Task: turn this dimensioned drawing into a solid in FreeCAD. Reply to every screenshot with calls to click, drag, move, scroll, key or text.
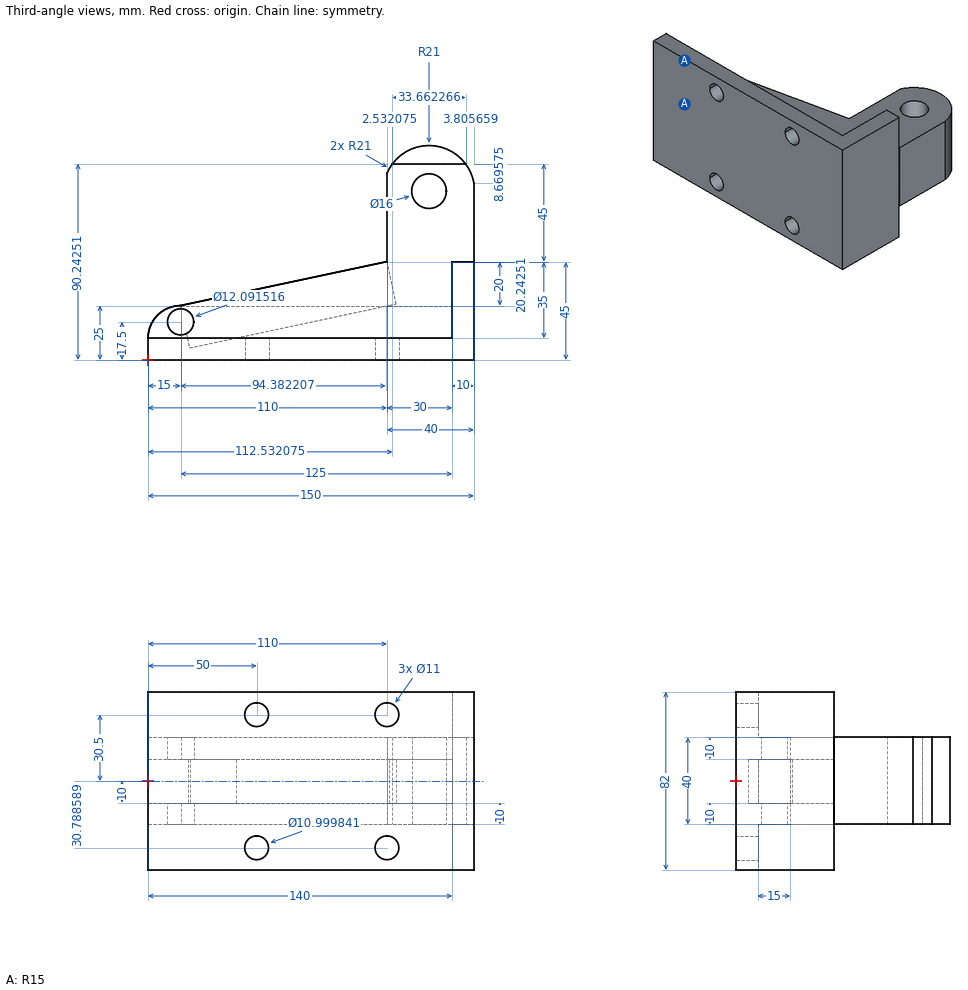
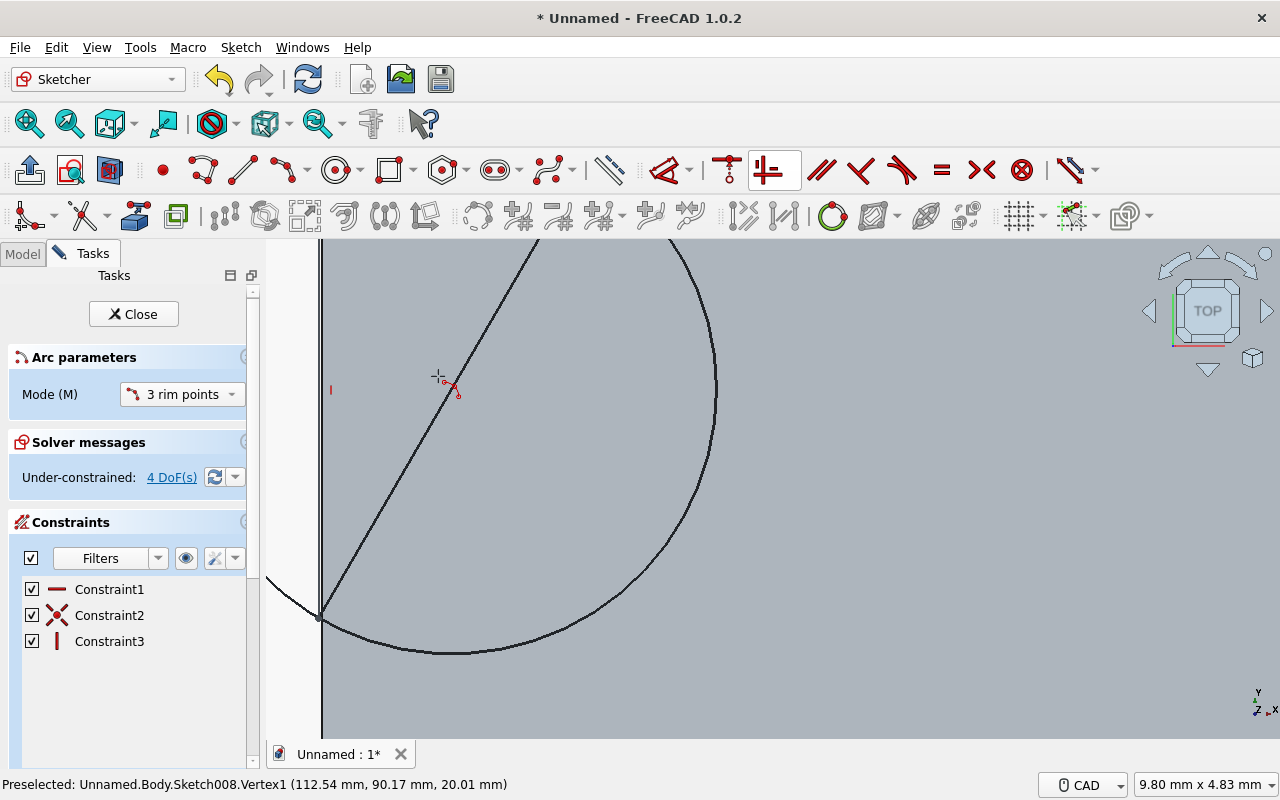
click(439, 374)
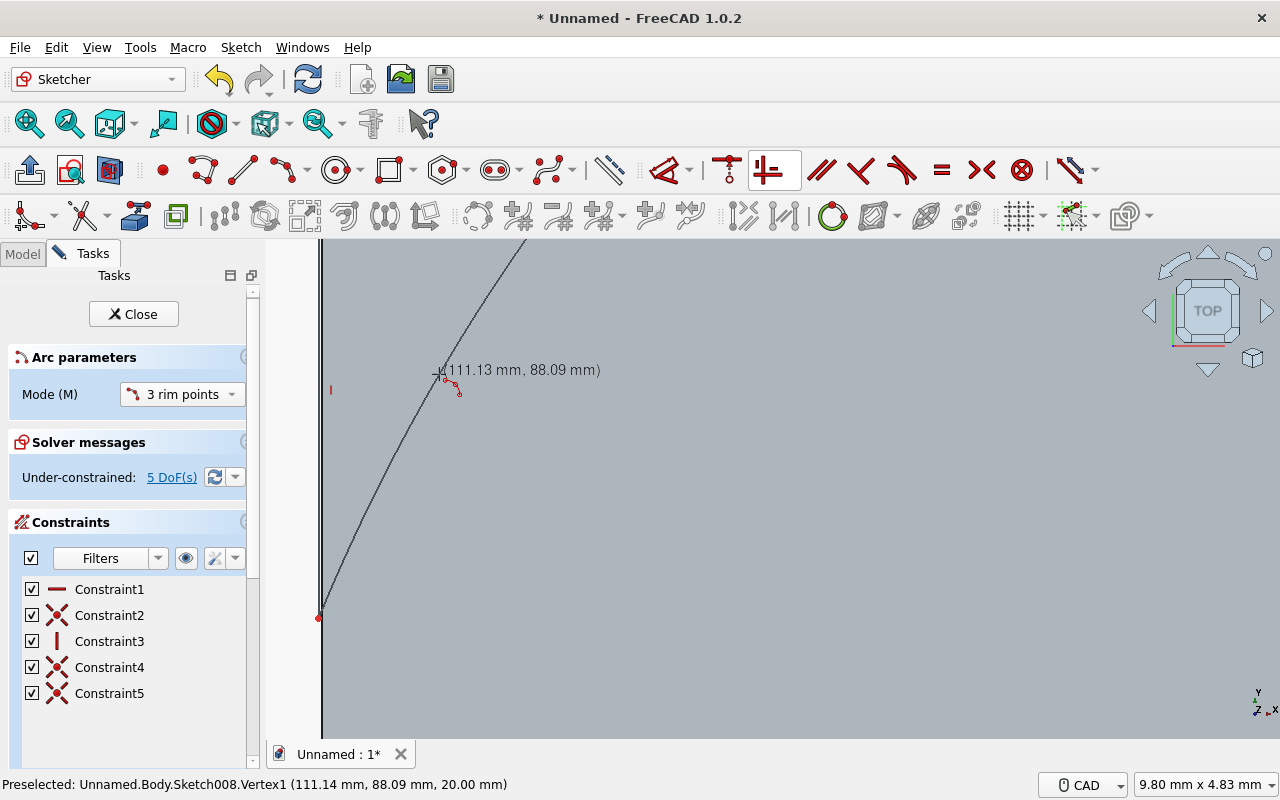
click(204, 170)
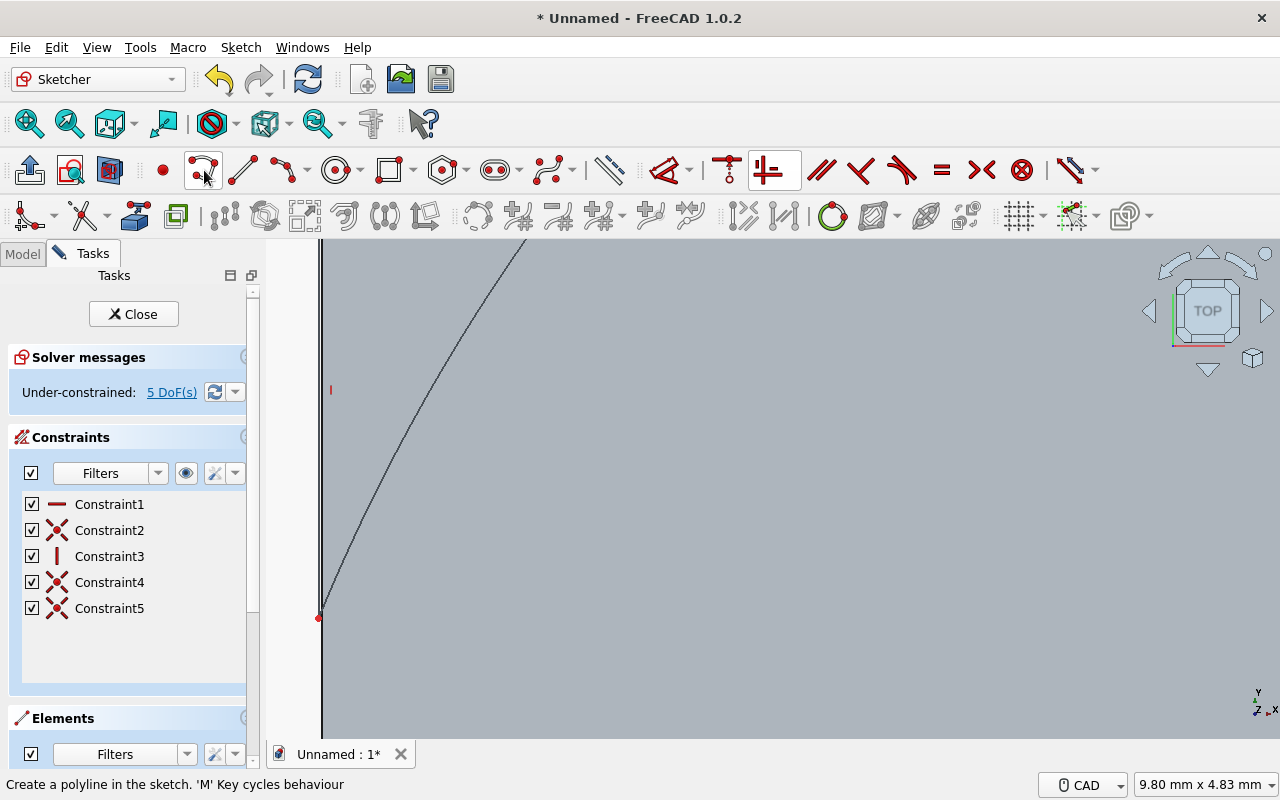
scroll(440, 375, down, 10)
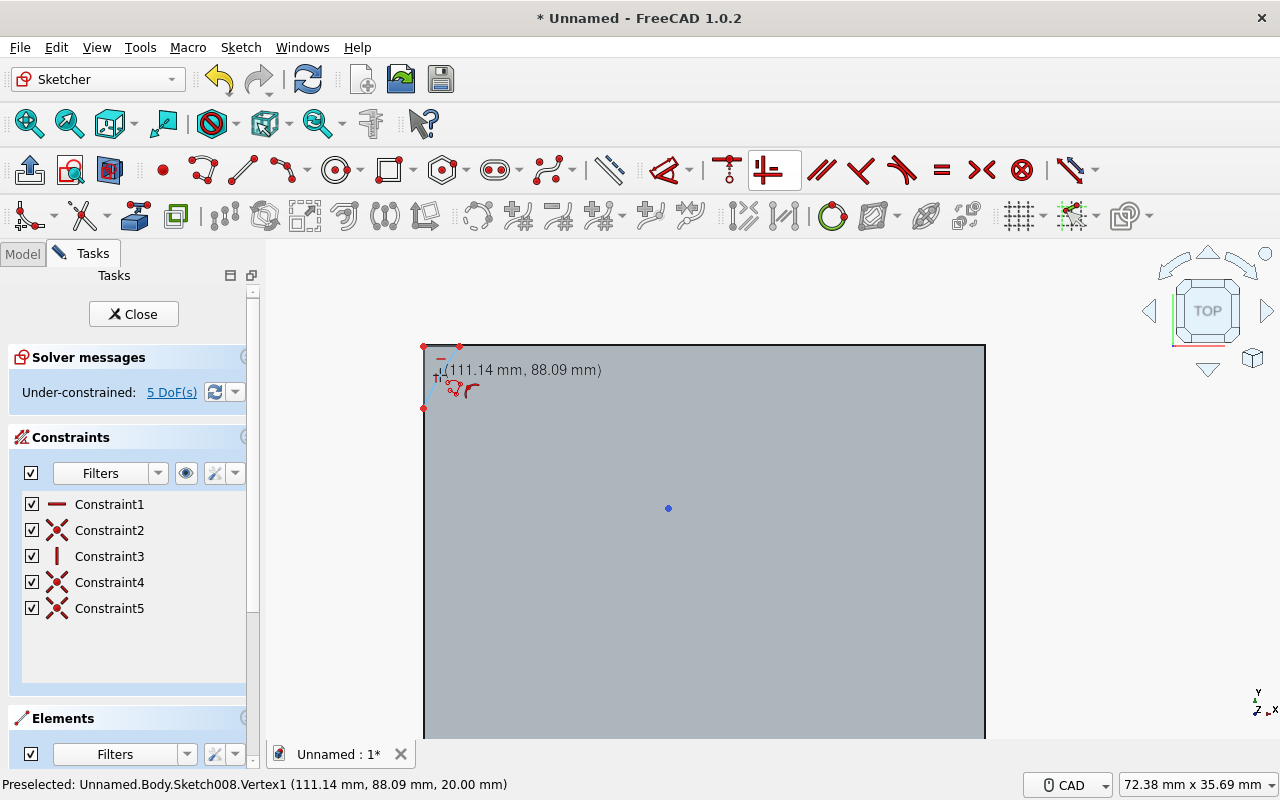
click(985, 467)
click(985, 345)
click(931, 345)
right_click(931, 345)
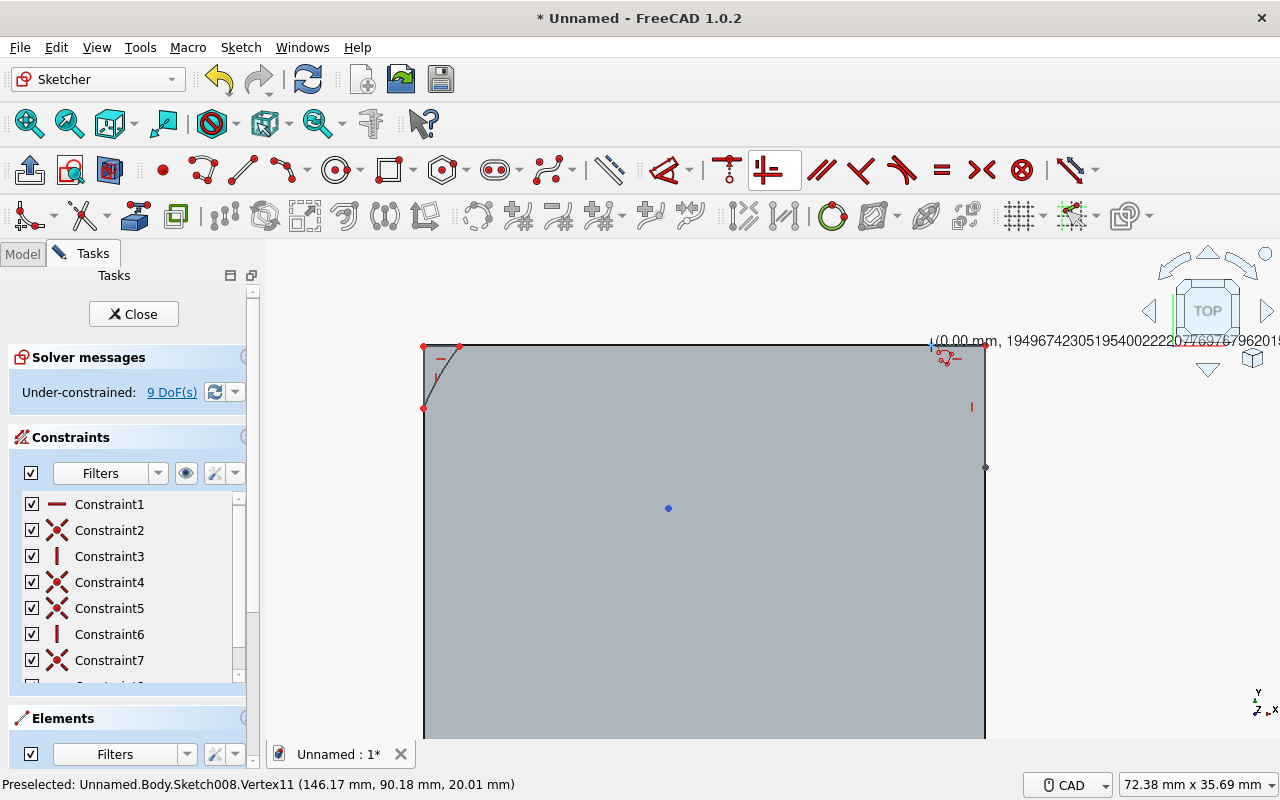
click(284, 170)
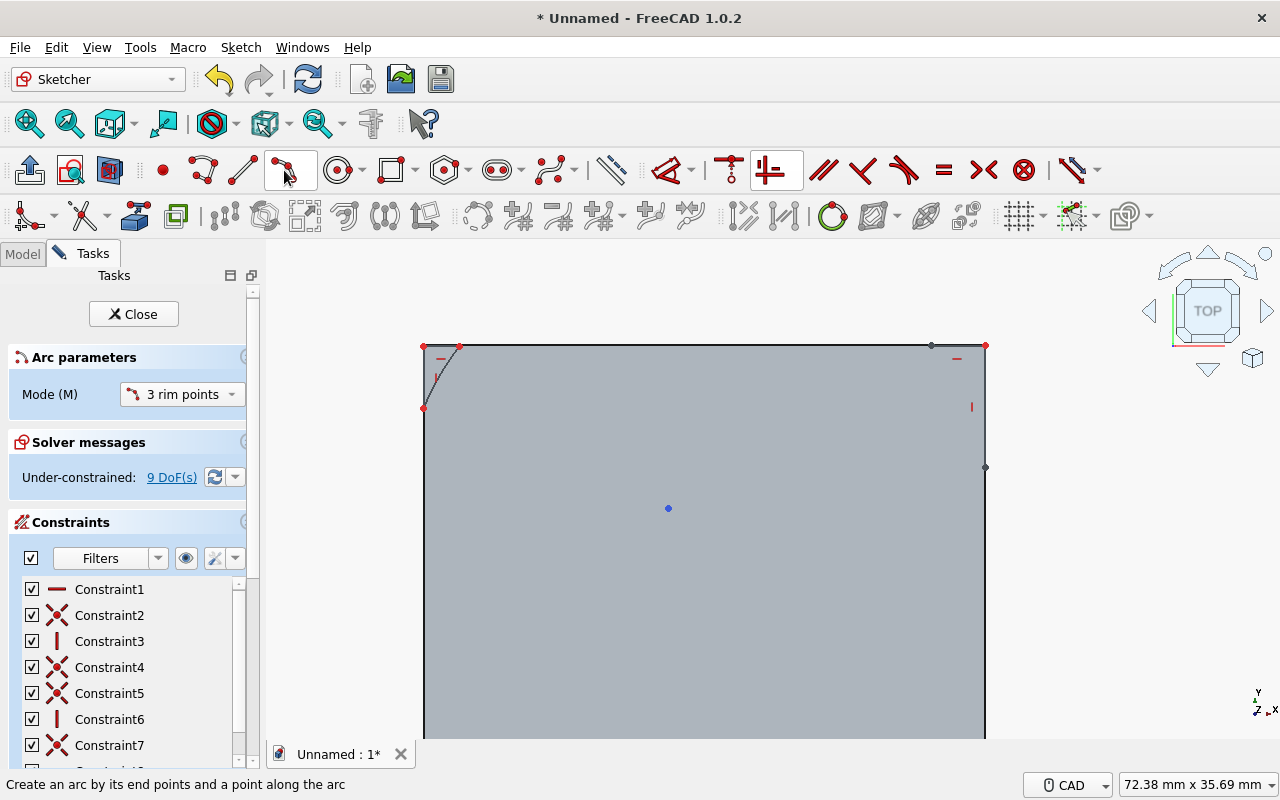
click(931, 346)
click(985, 468)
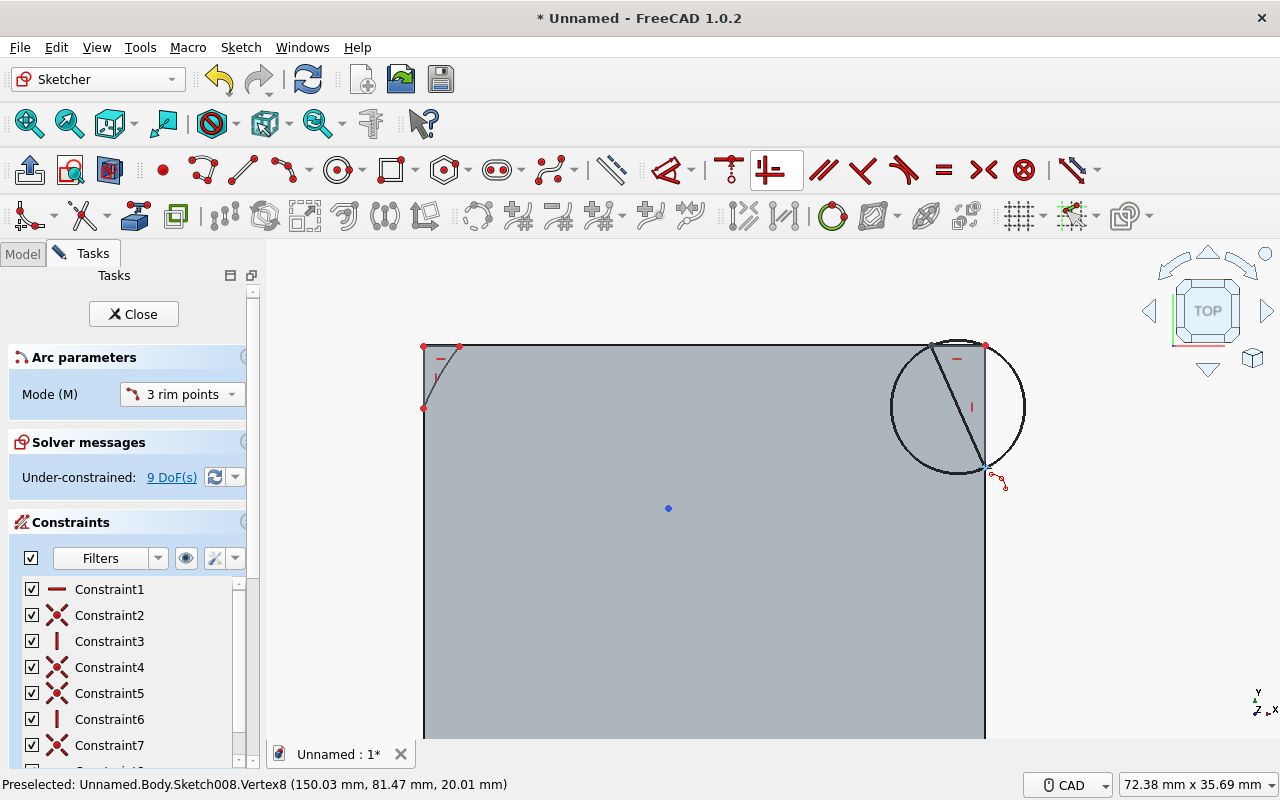
scroll(965, 403, up, 4)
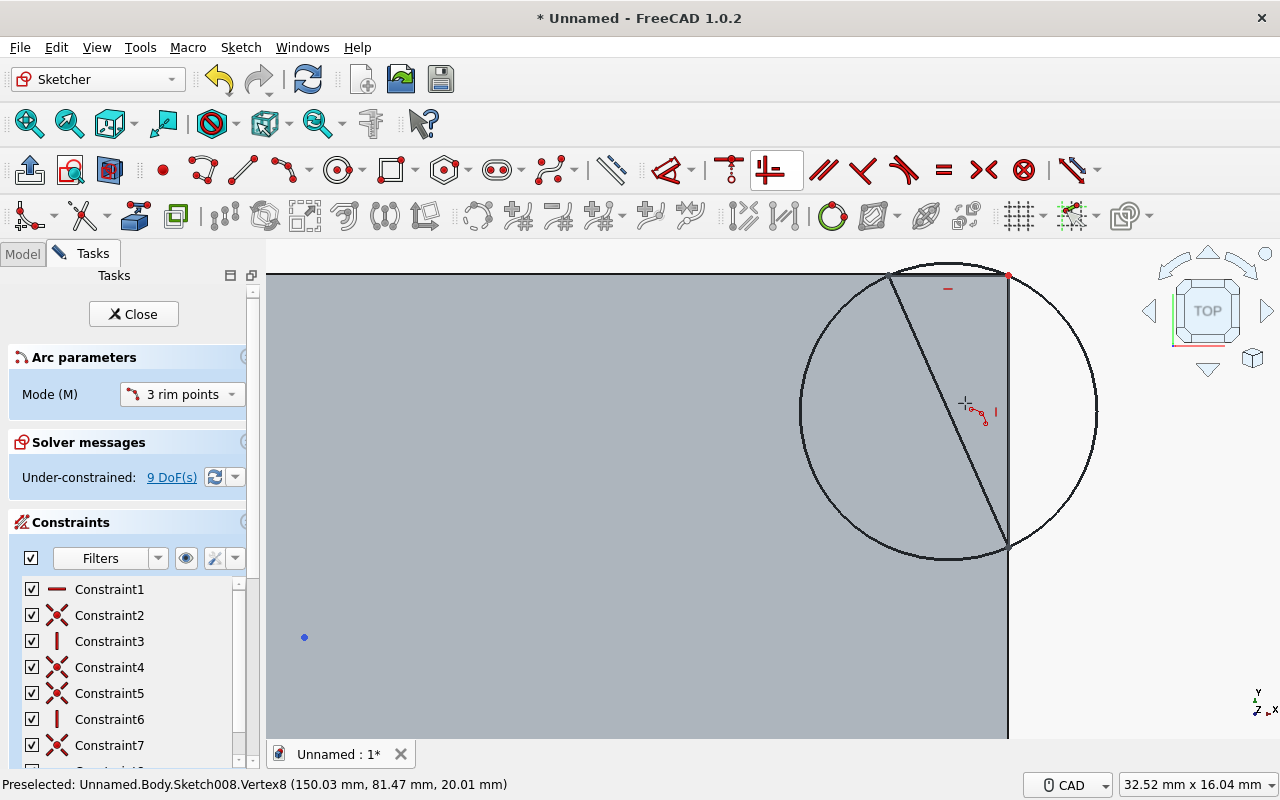
click(964, 402)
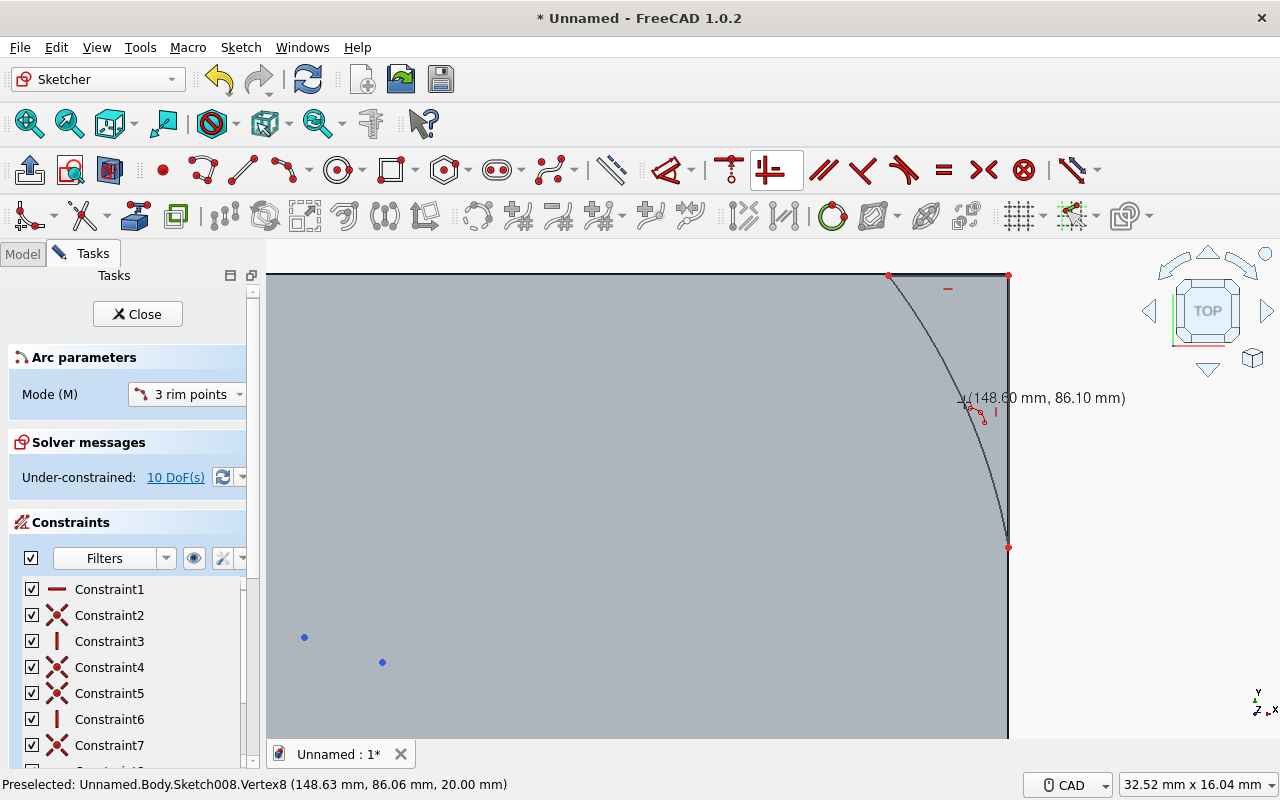
key(g)
key(c)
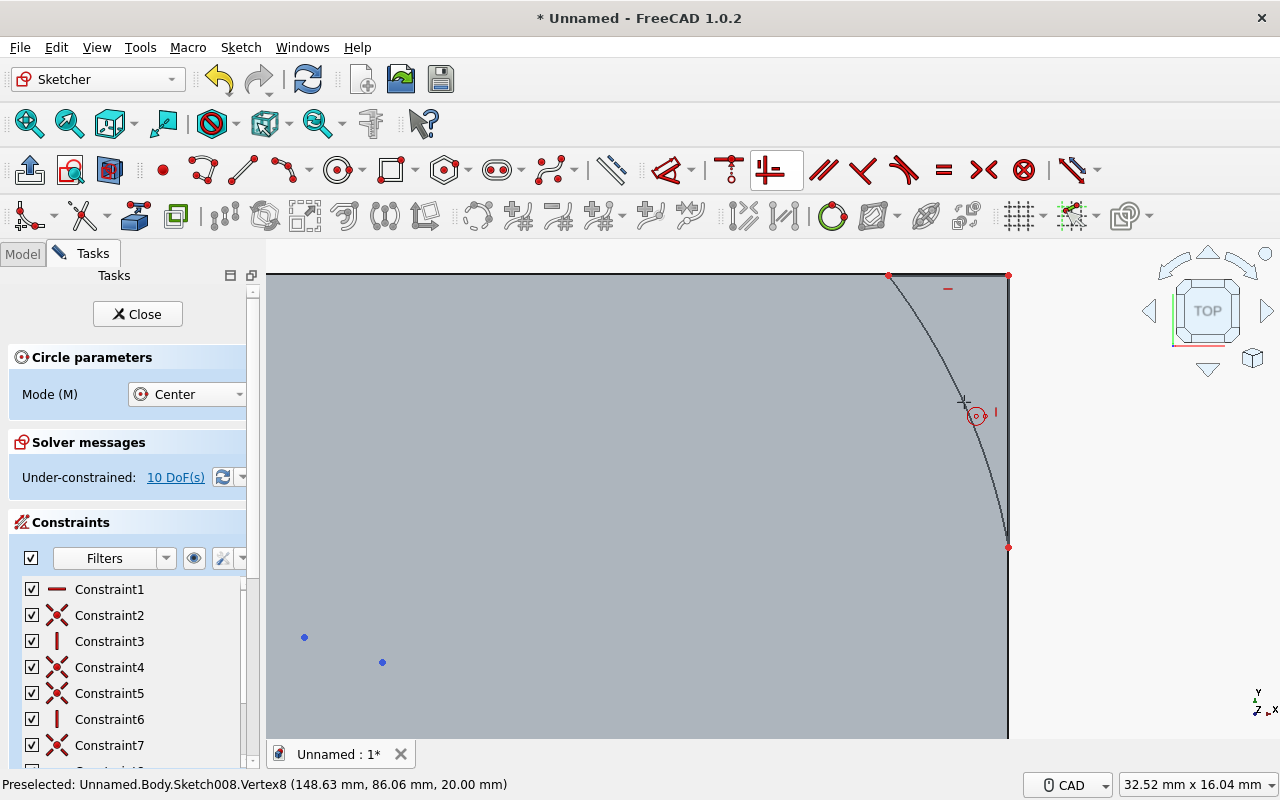
click(364, 665)
move(541, 489)